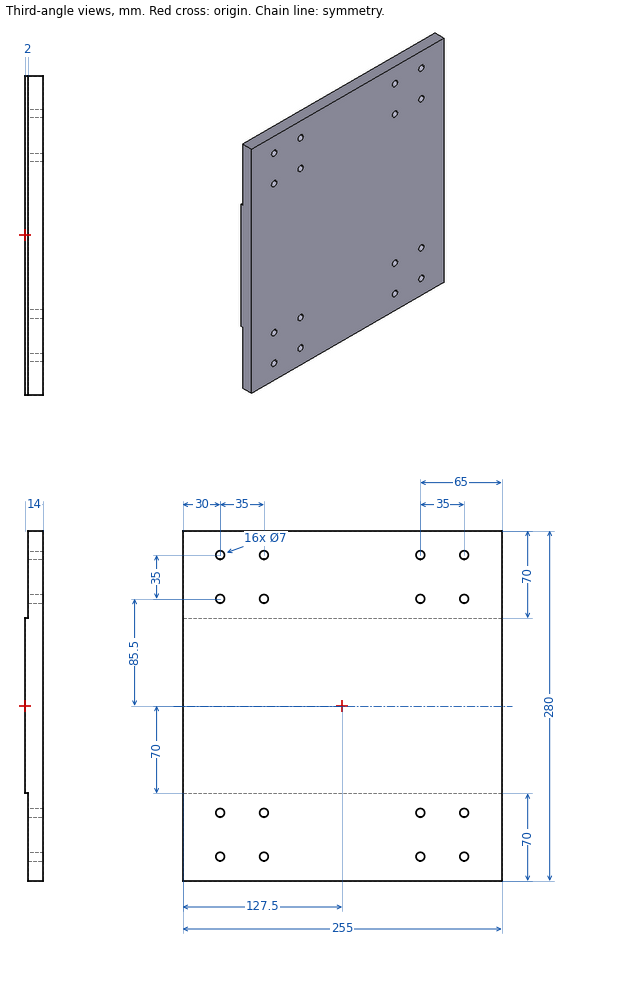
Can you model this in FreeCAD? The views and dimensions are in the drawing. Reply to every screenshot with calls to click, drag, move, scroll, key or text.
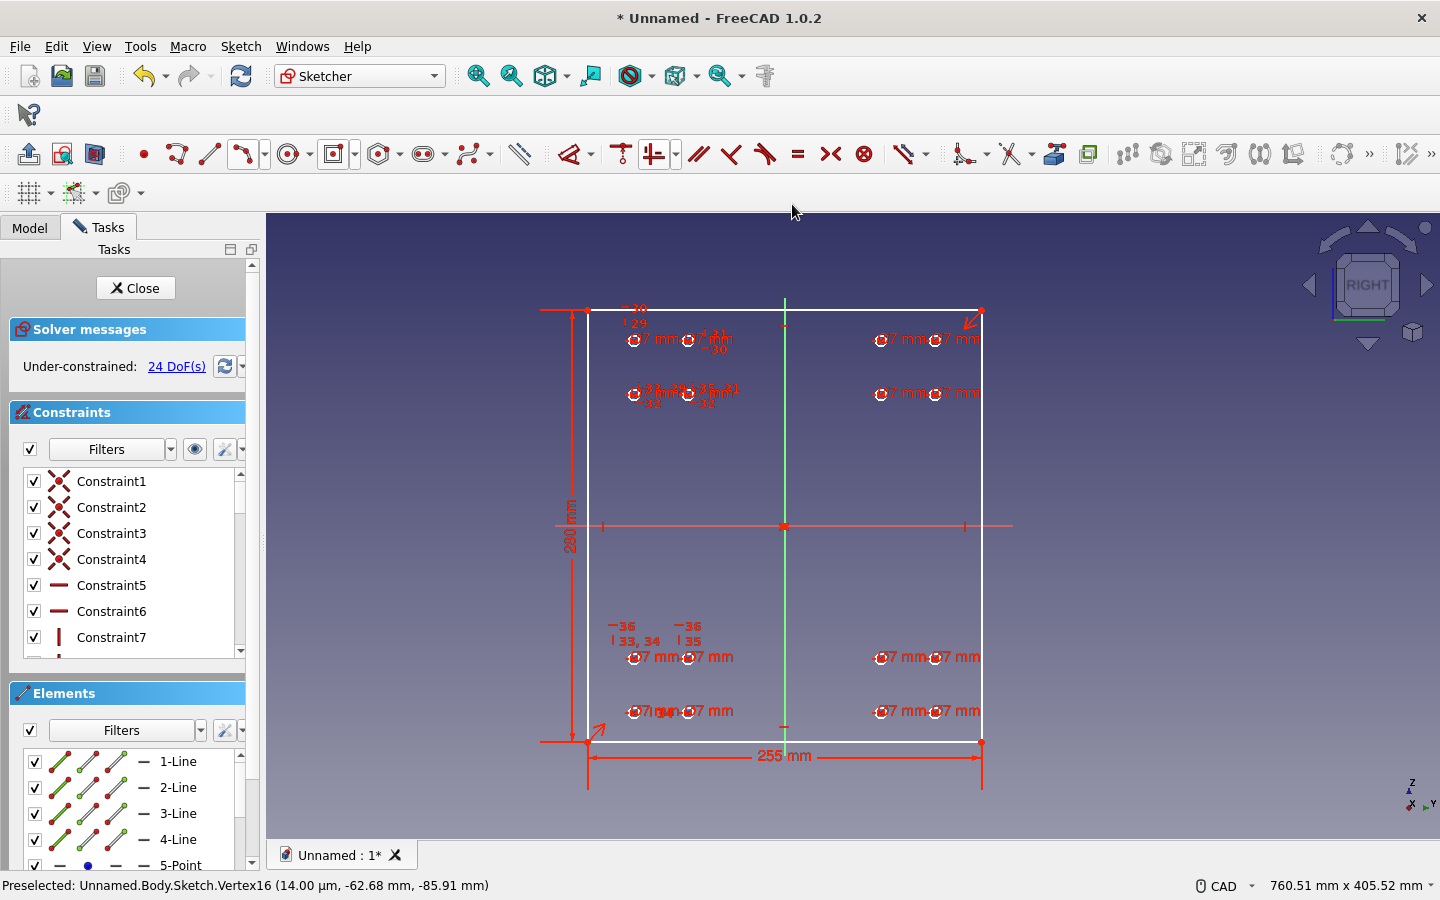
click(688, 659)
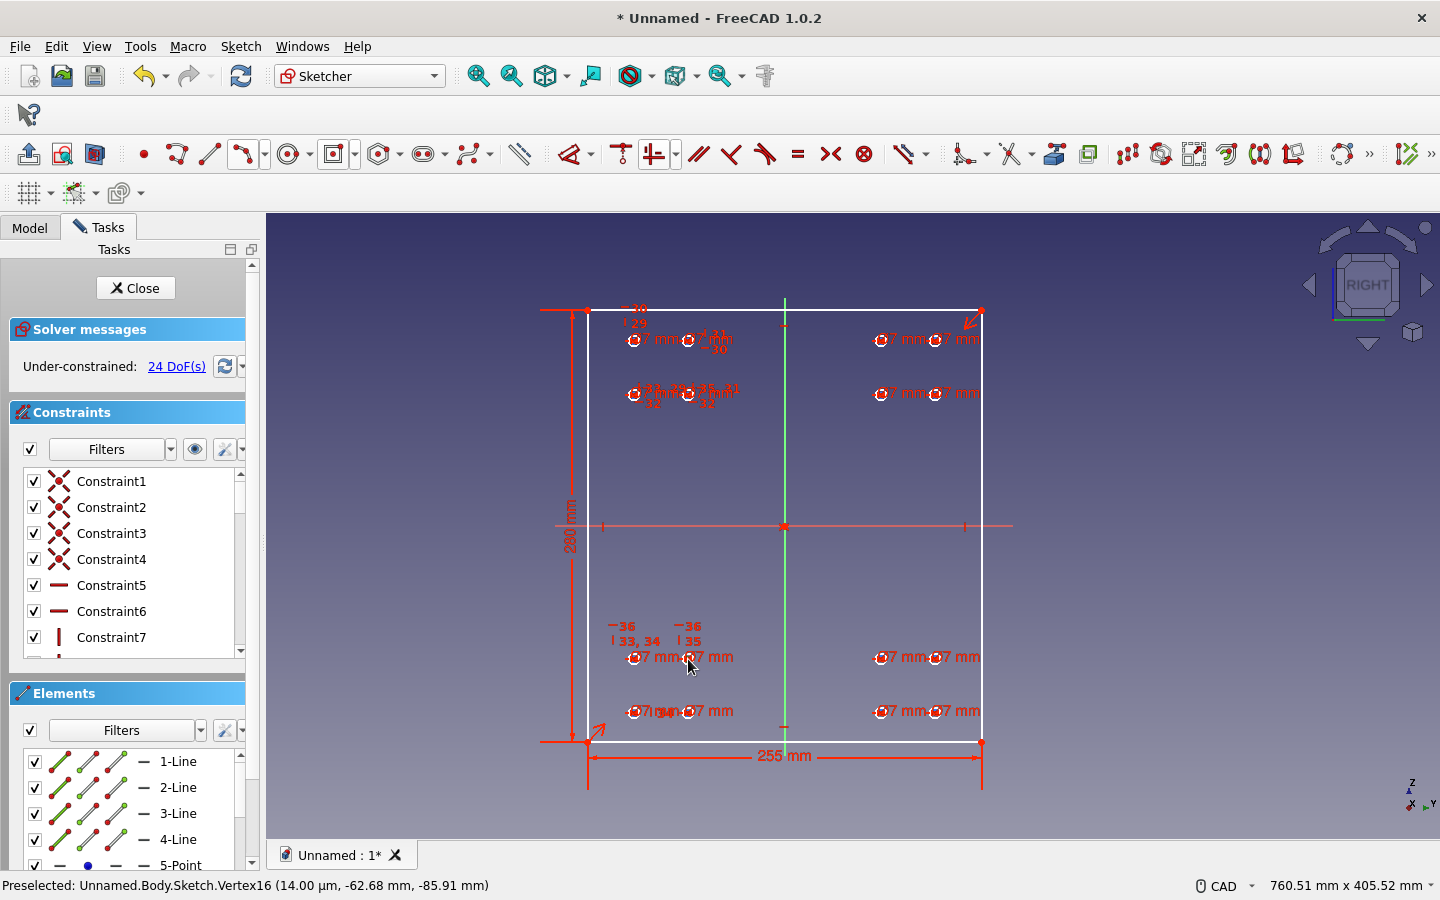
click(688, 713)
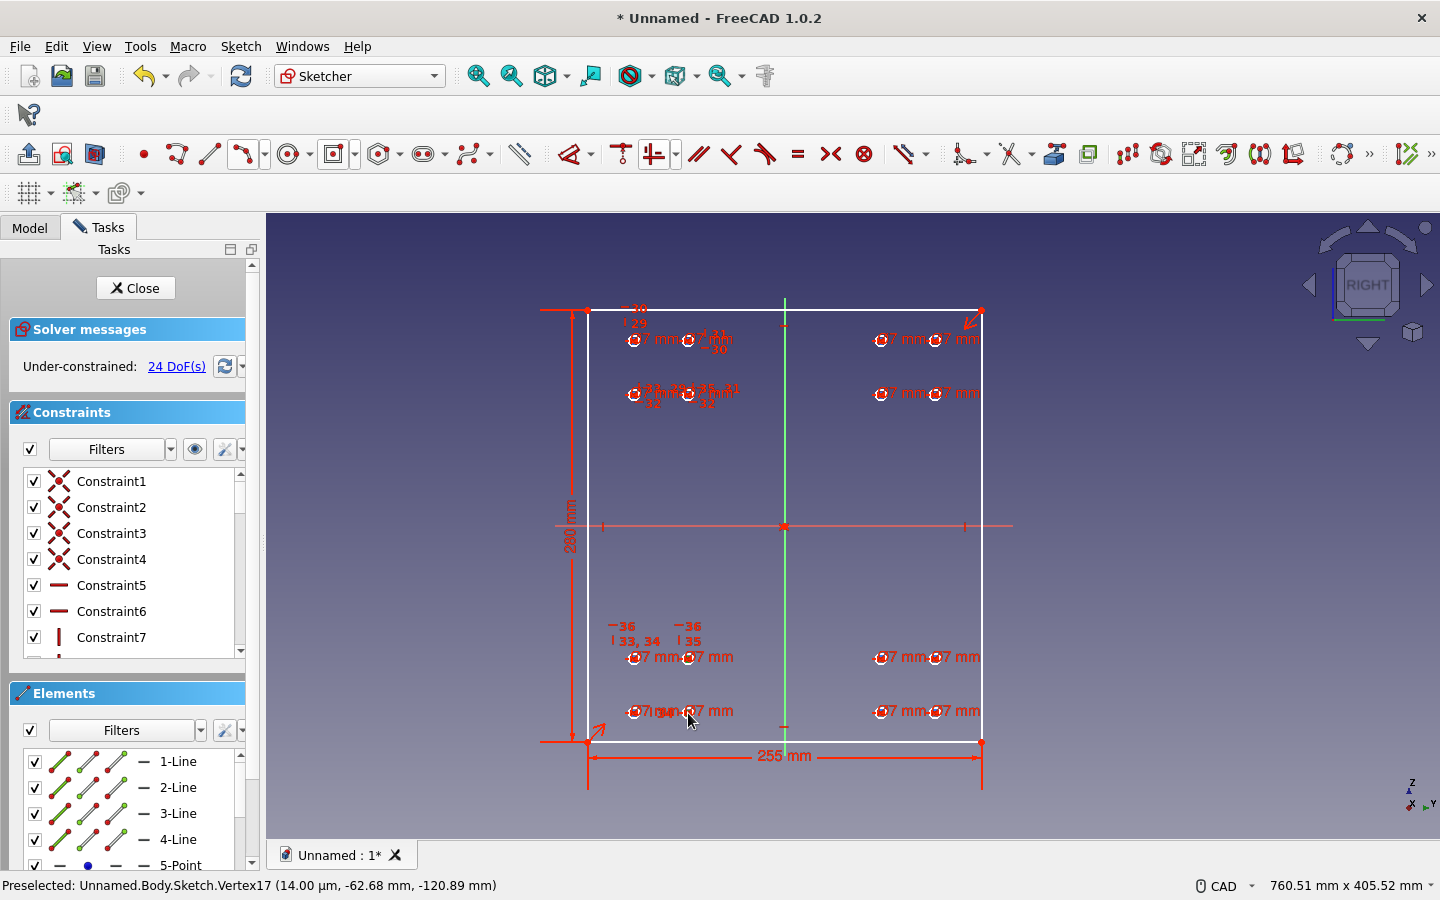
click(676, 154)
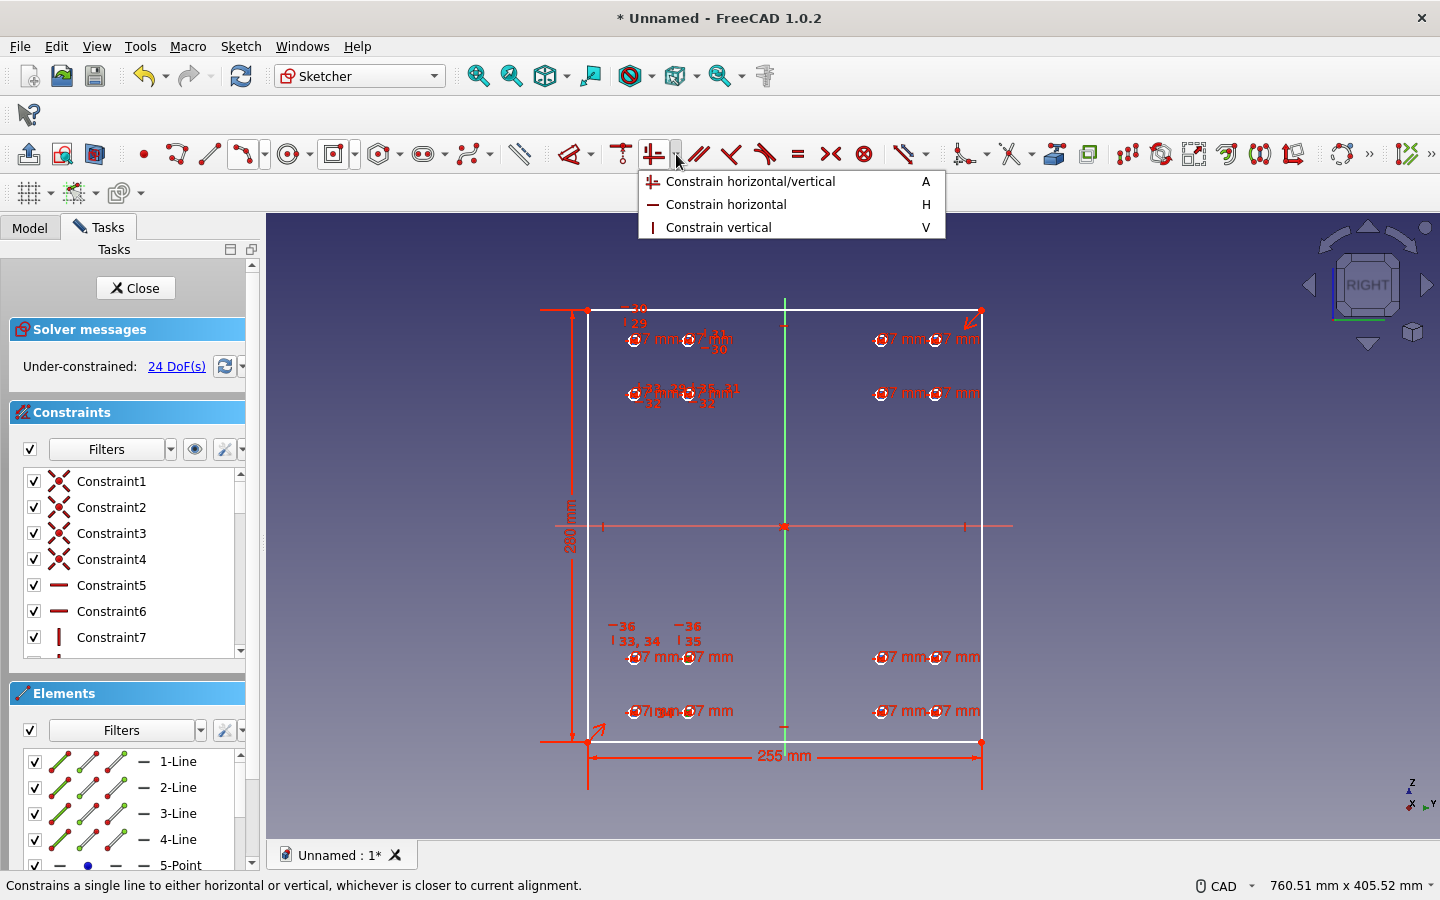
click(792, 228)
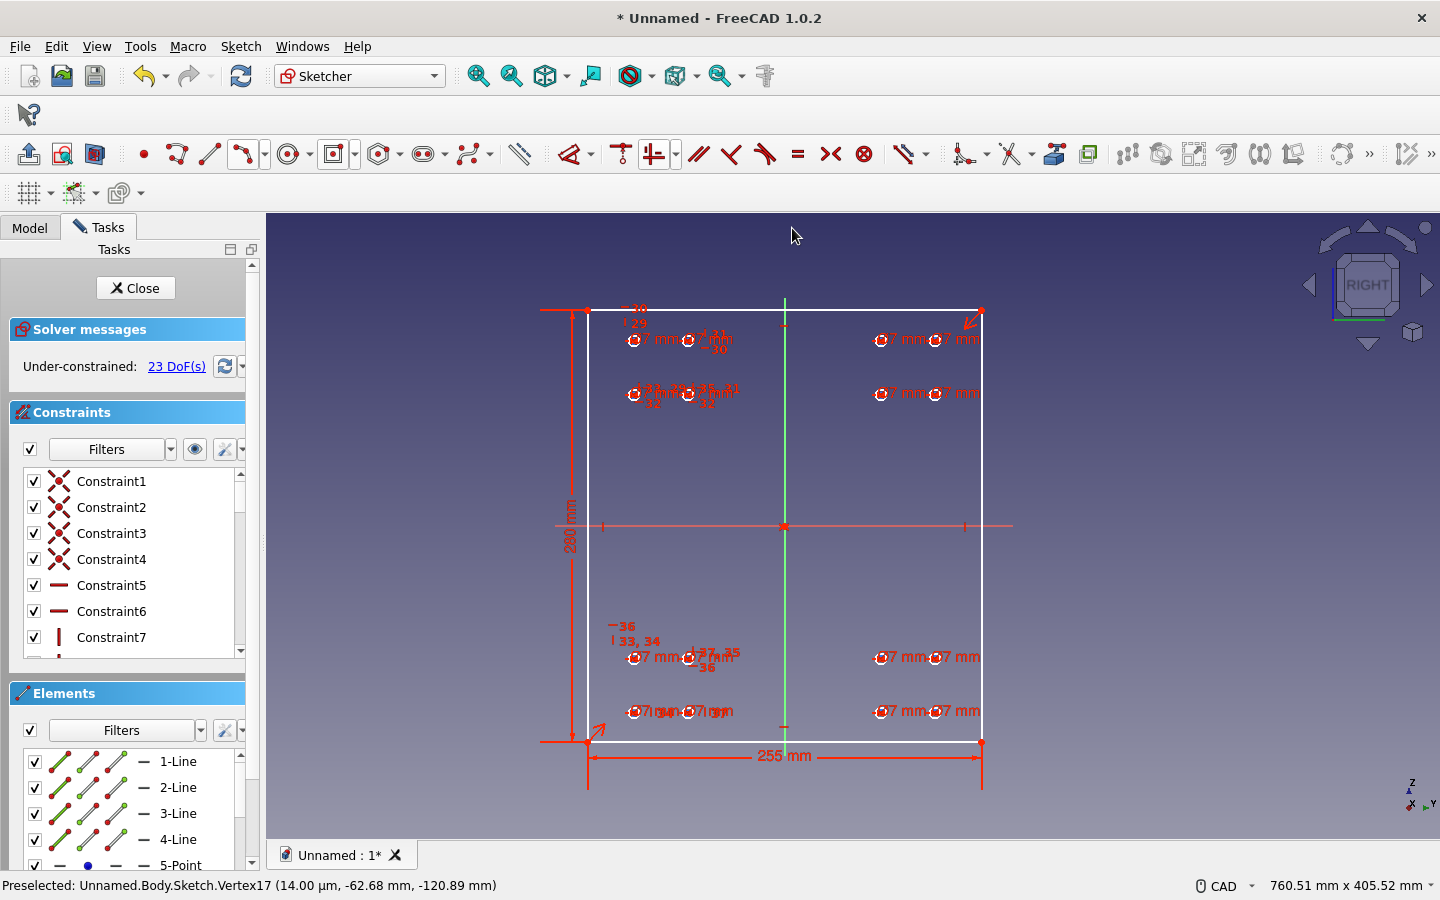
click(634, 713)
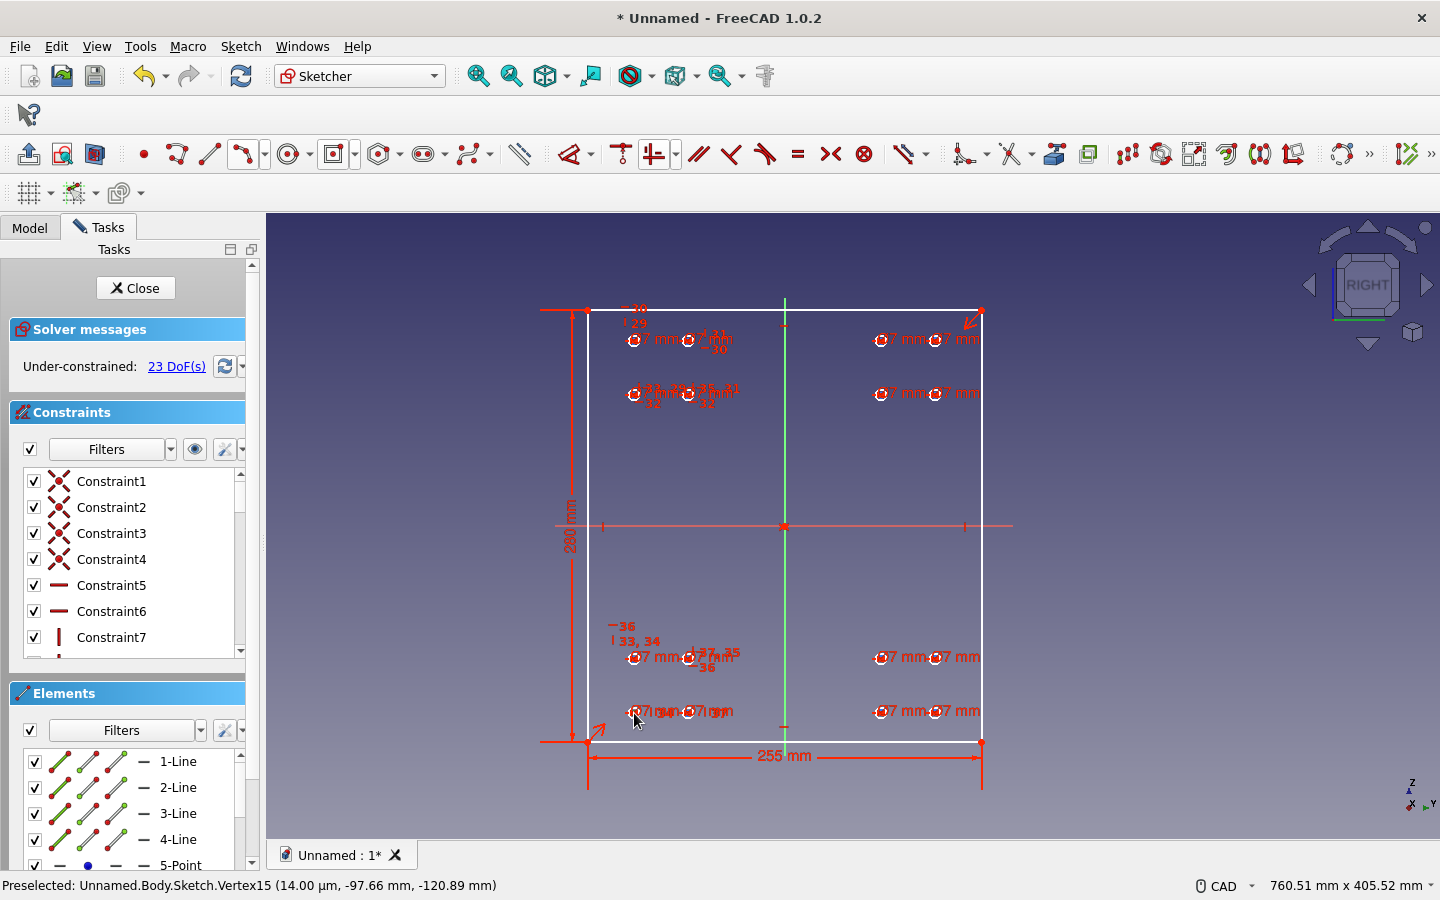
click(688, 713)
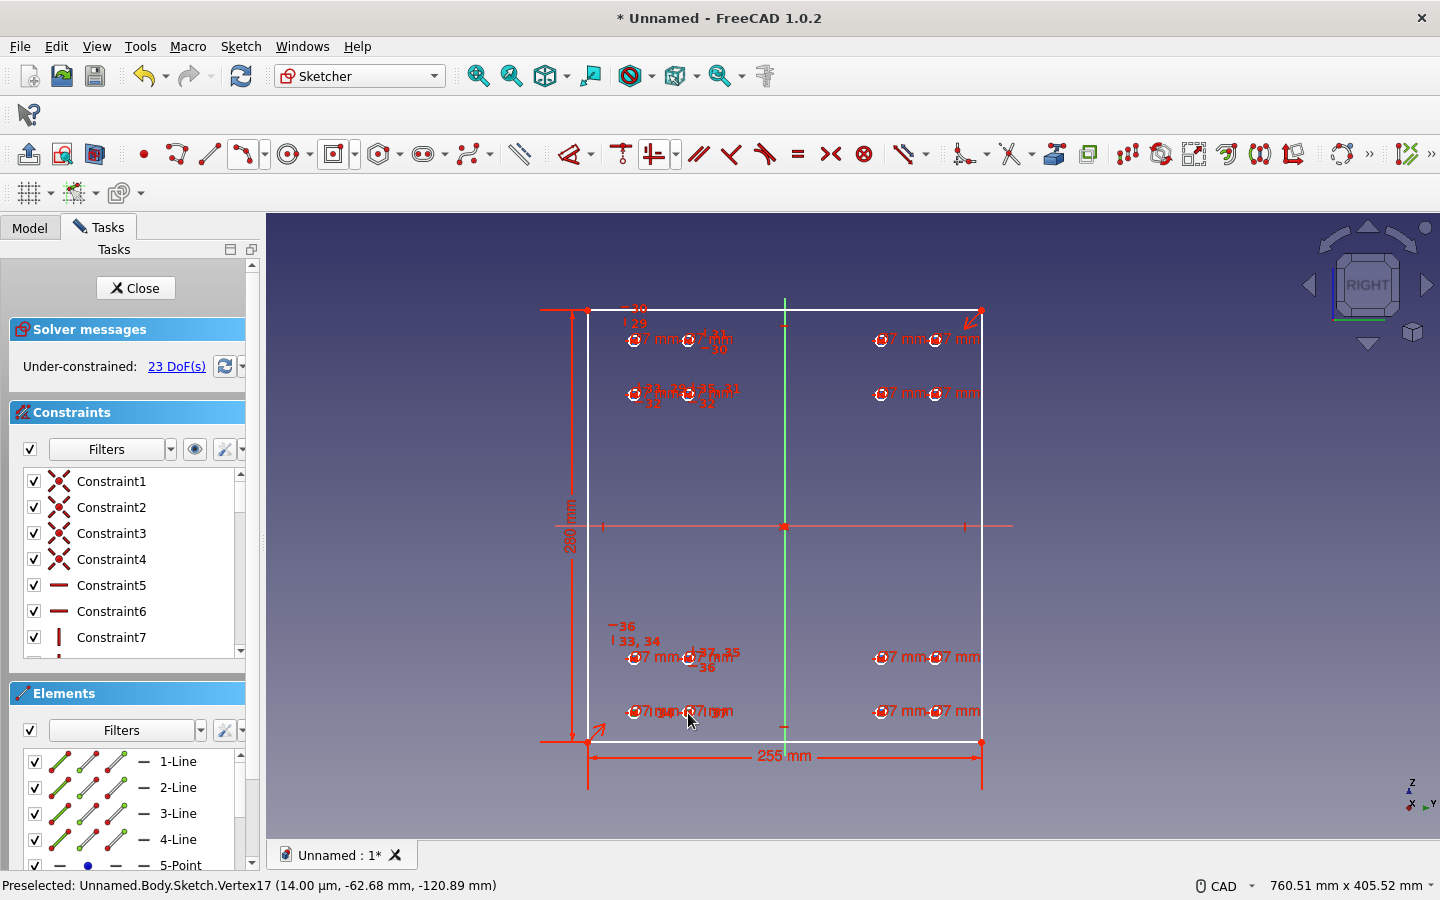
key(h)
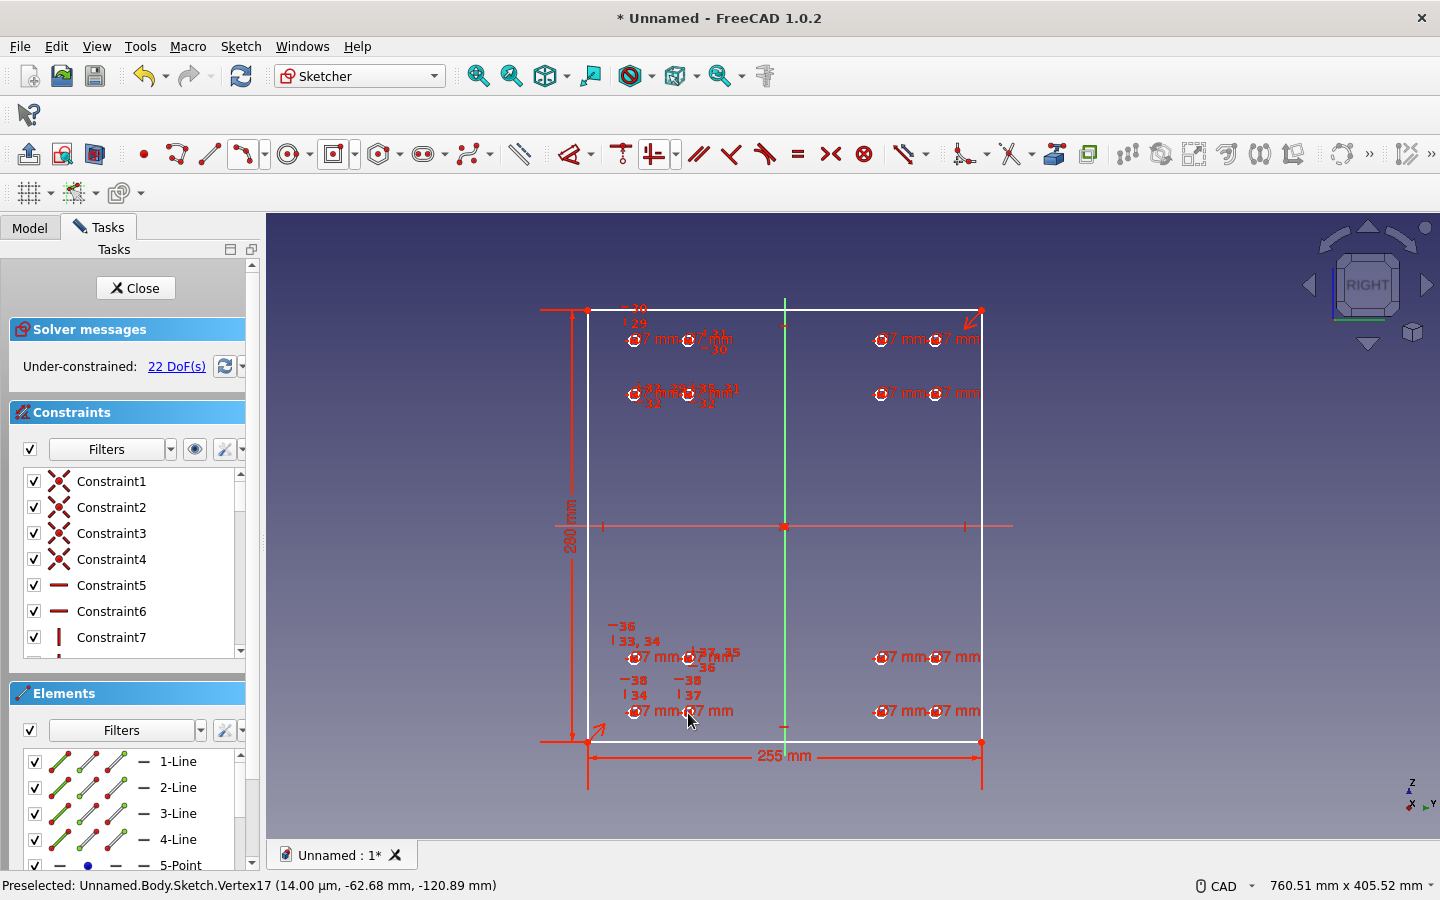
click(688, 341)